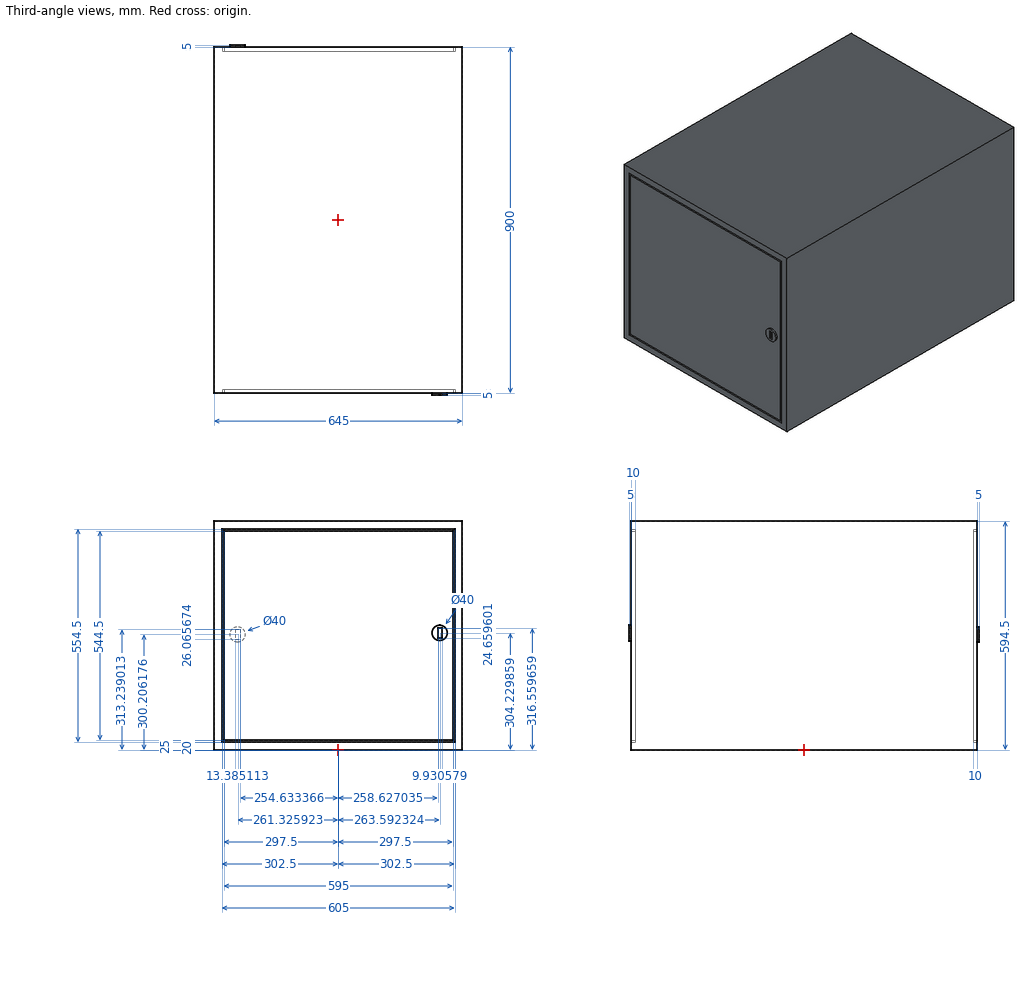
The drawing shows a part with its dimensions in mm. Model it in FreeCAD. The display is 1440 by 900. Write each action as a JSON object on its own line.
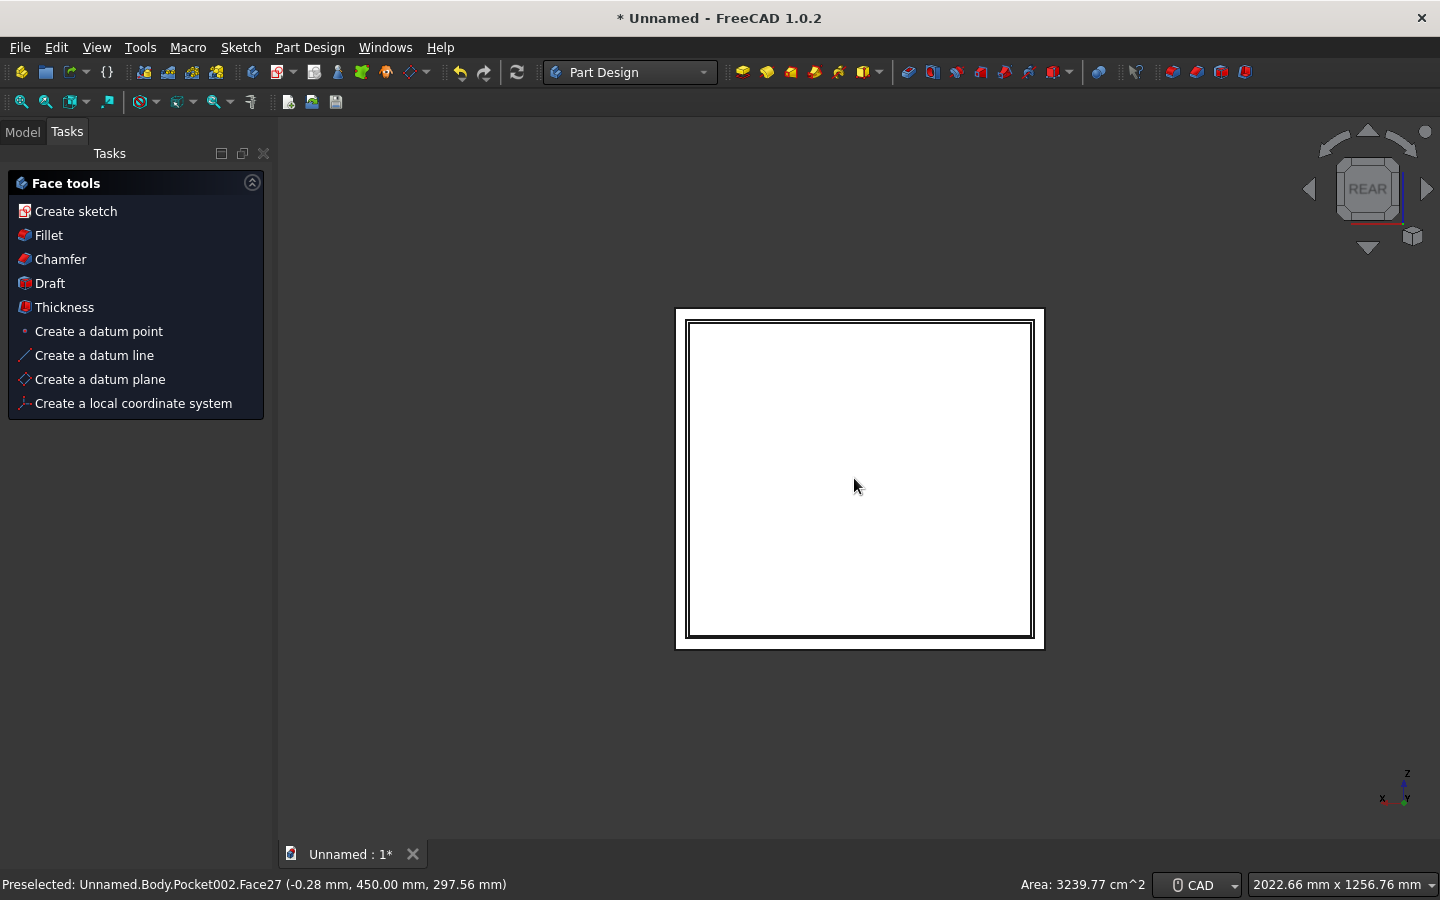
{"action": "left_click", "coordinate": [278, 72]}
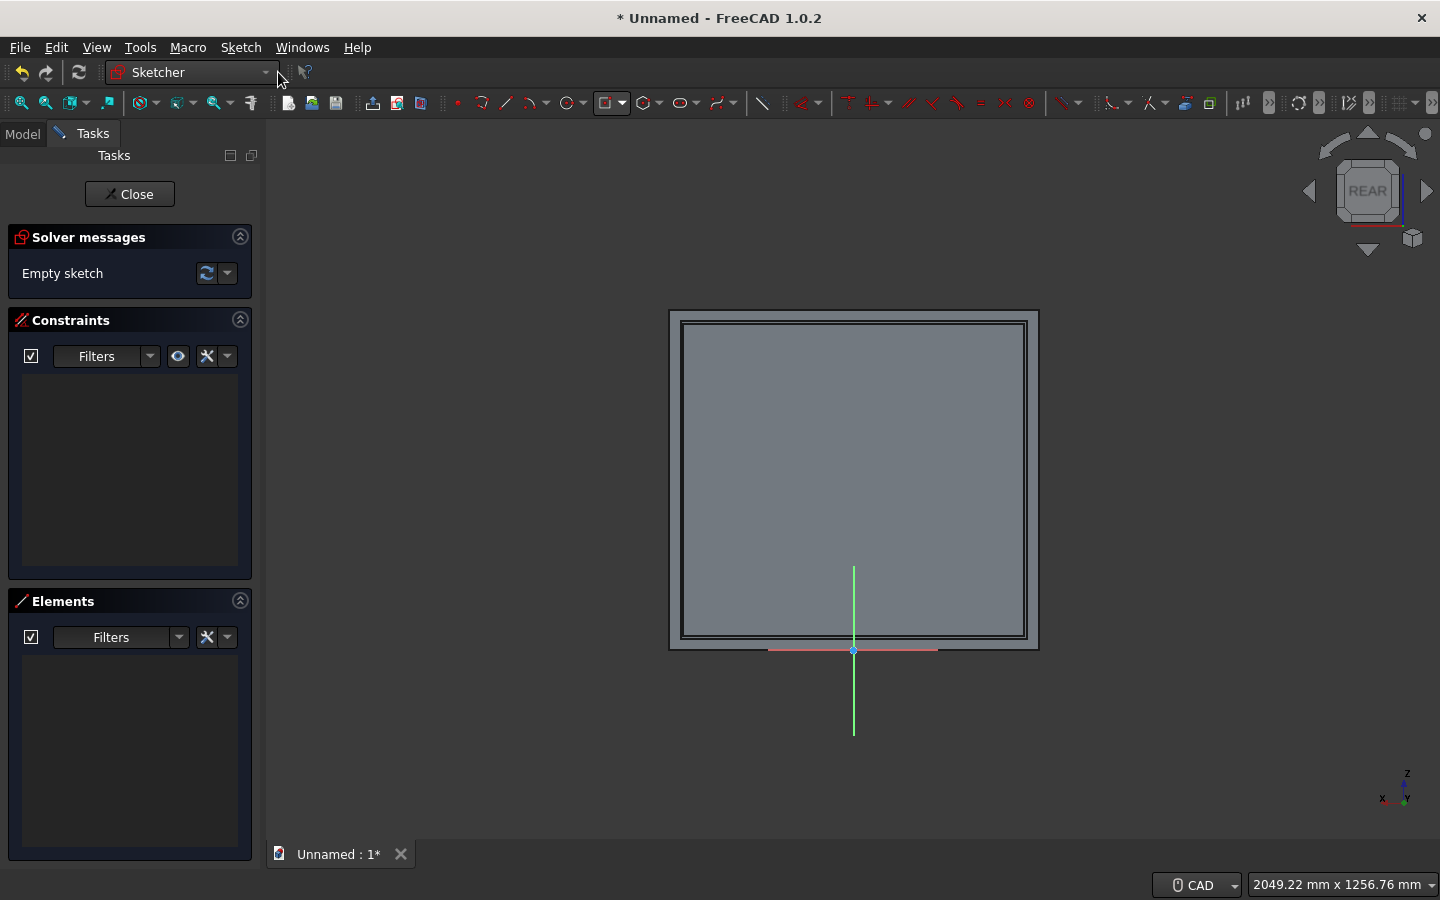
{"action": "scroll", "coordinate": [1015, 478], "scroll_direction": "up", "scroll_amount": 15}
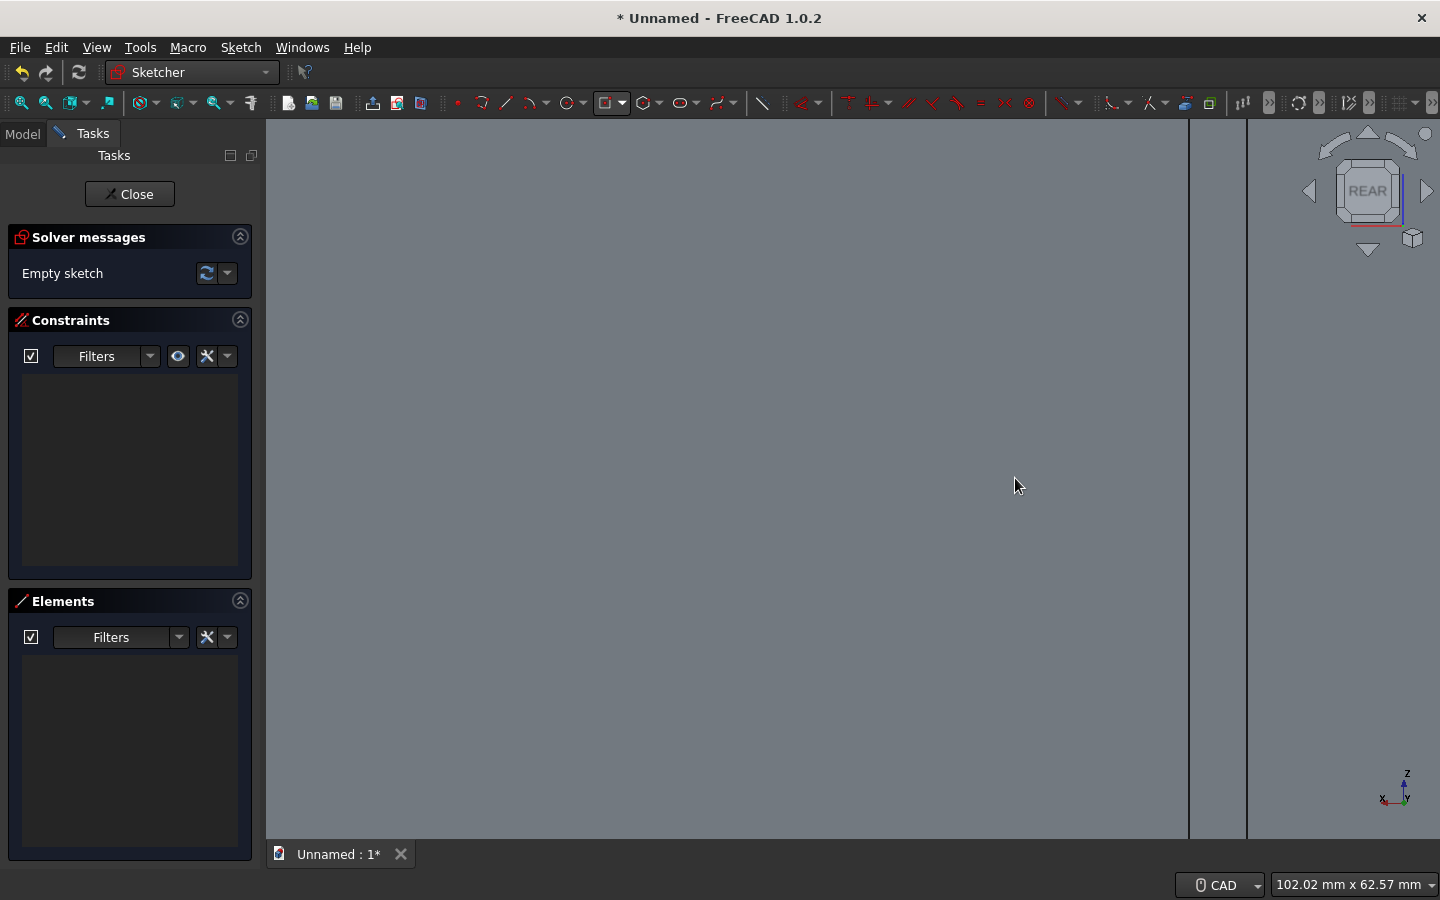
{"action": "left_click", "coordinate": [568, 104]}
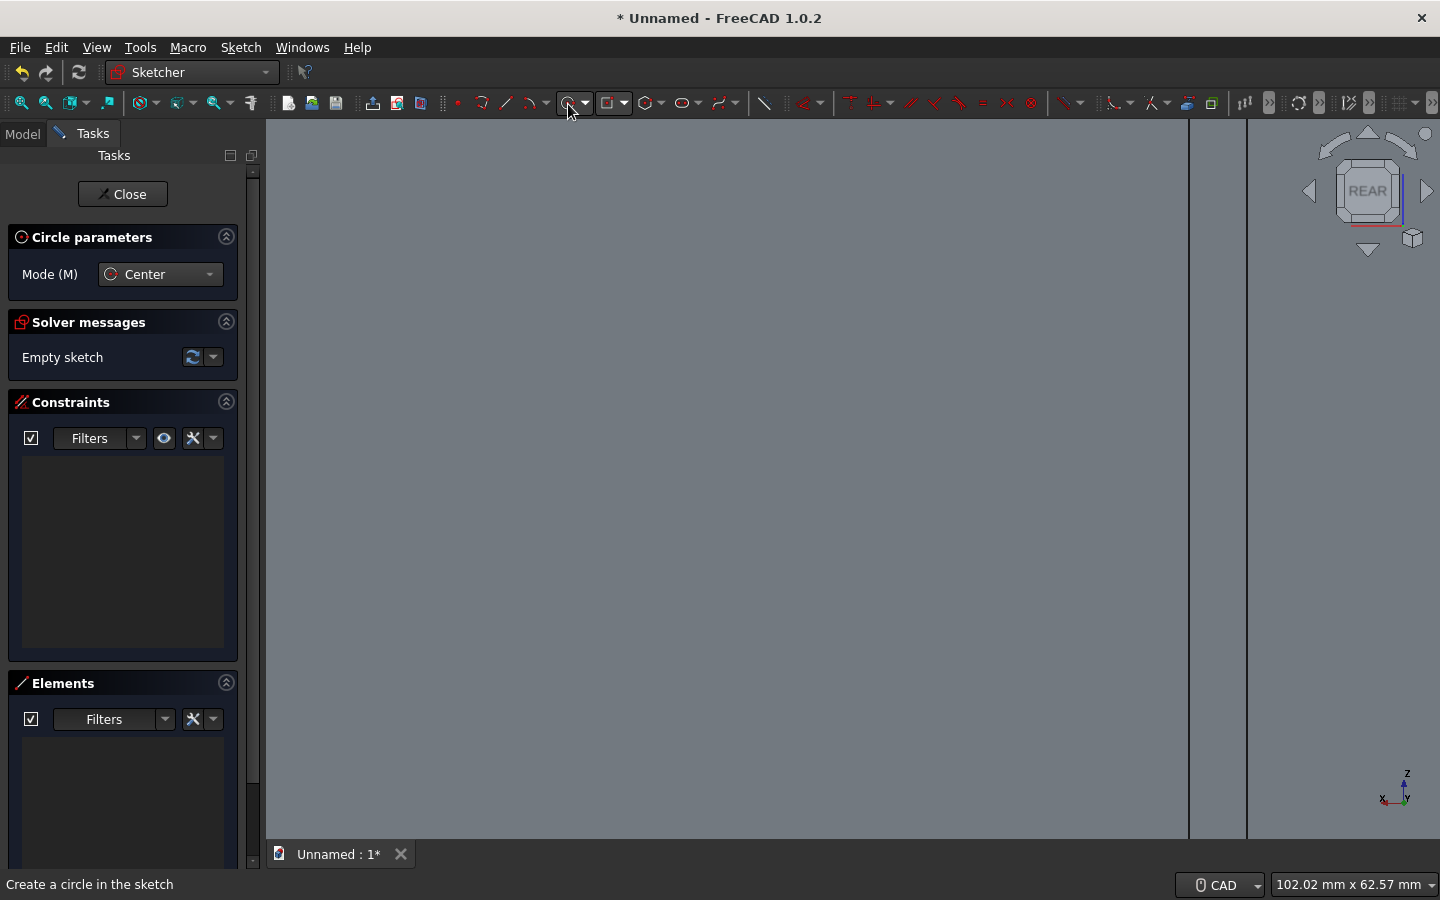
{"action": "left_click", "coordinate": [773, 478]}
{"action": "left_click", "coordinate": [936, 315]}
{"action": "key", "text": "Escape"}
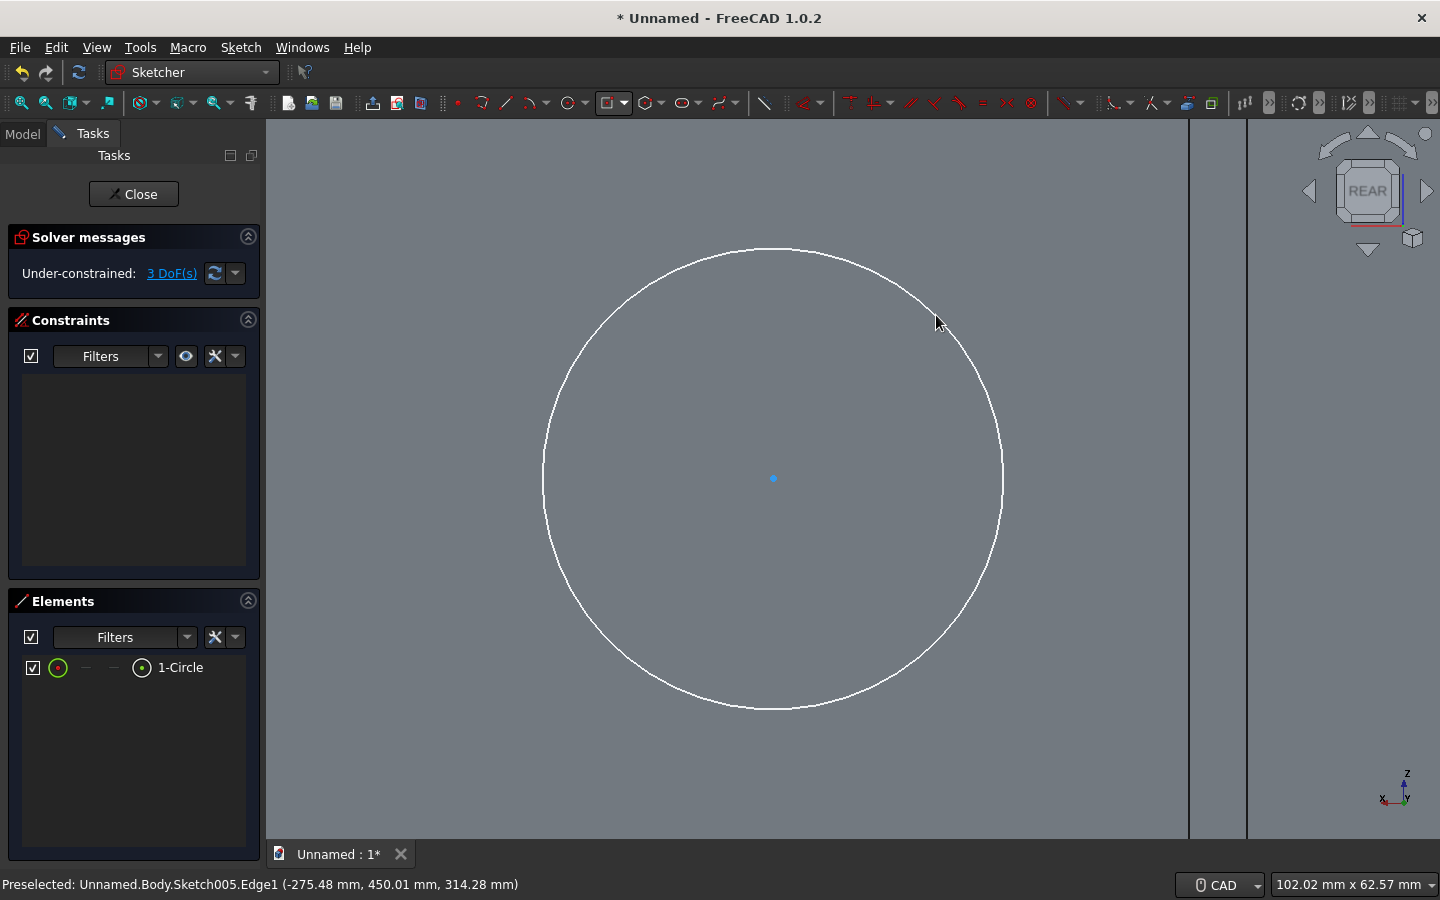
{"action": "left_click", "coordinate": [804, 104]}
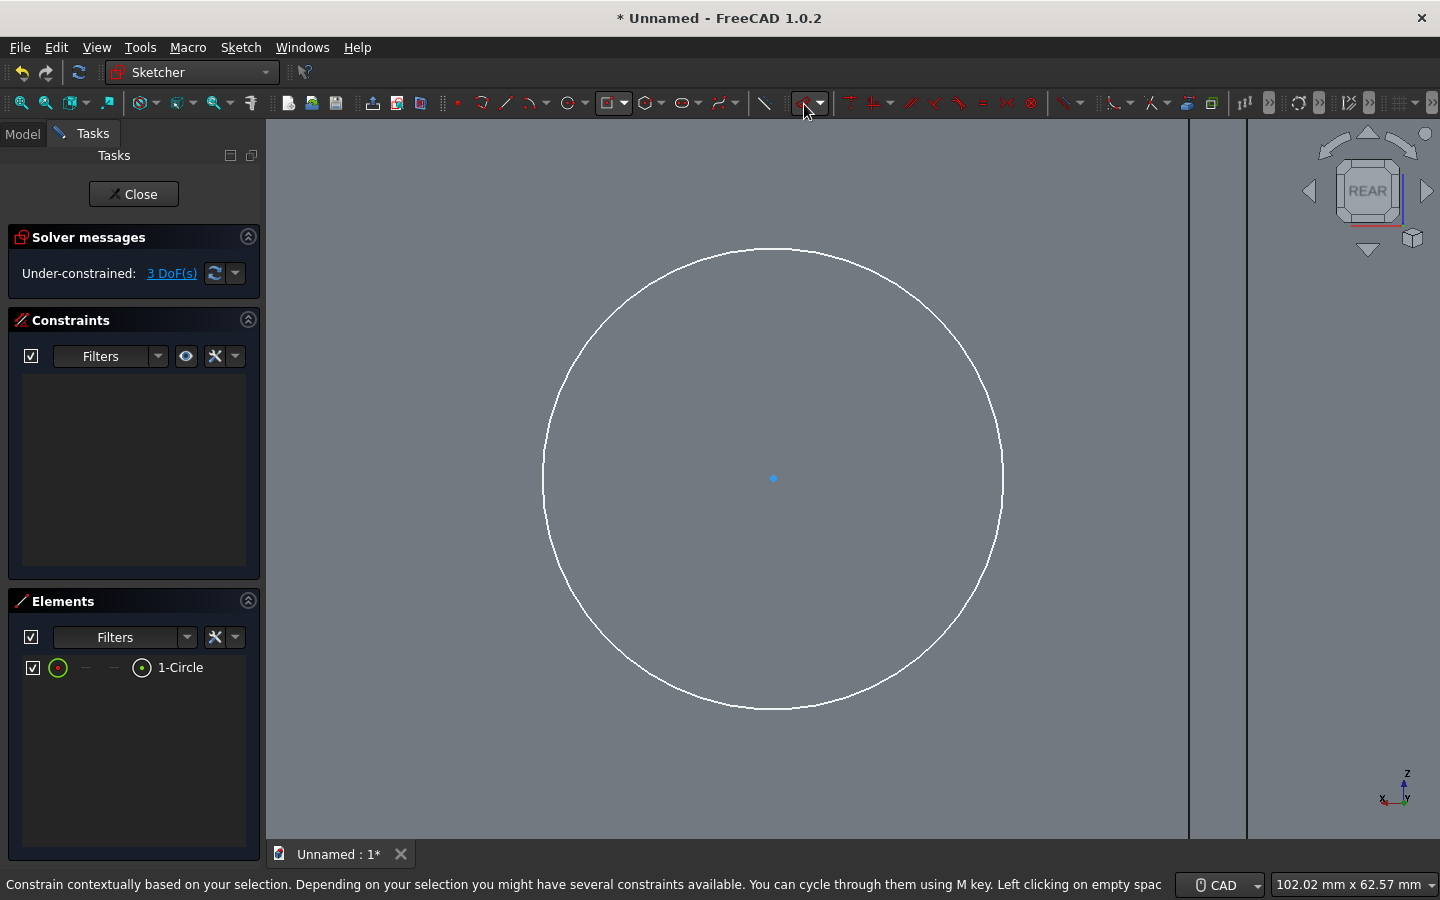
{"action": "left_click", "coordinate": [935, 315]}
{"action": "left_click", "coordinate": [957, 292]}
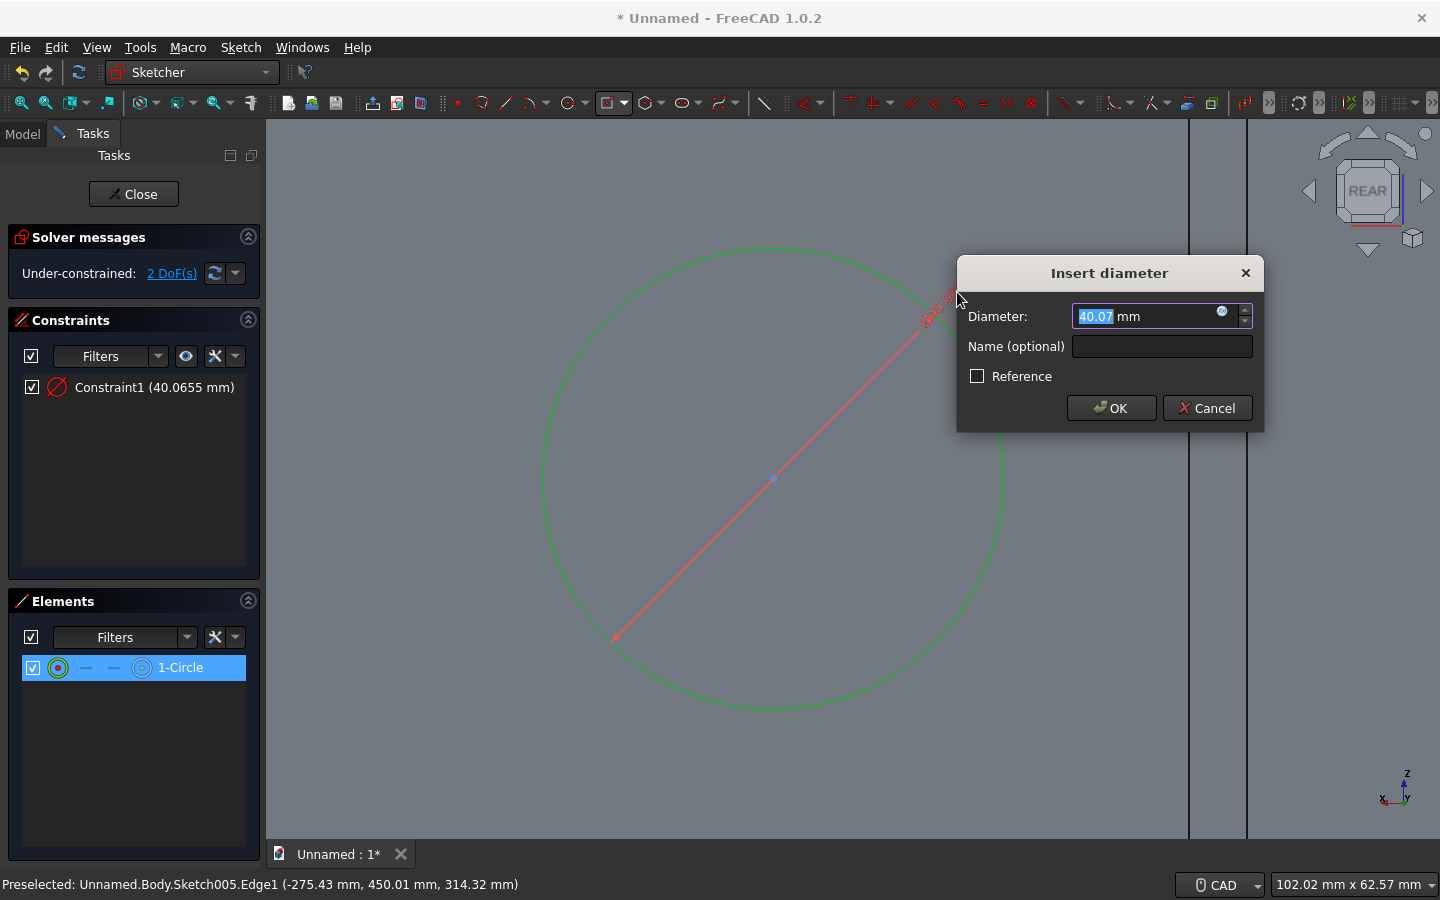
{"action": "type", "text": "40"}
{"action": "key", "text": "Return"}